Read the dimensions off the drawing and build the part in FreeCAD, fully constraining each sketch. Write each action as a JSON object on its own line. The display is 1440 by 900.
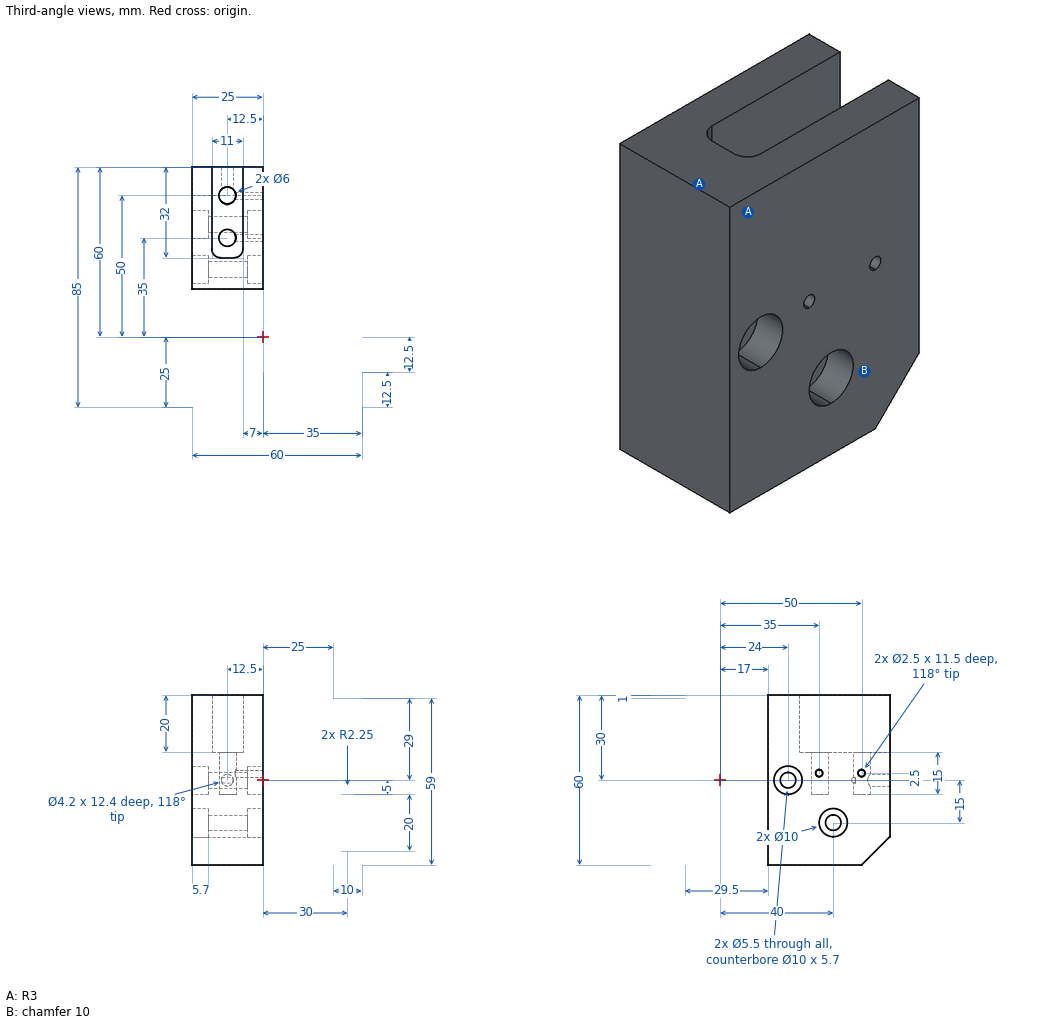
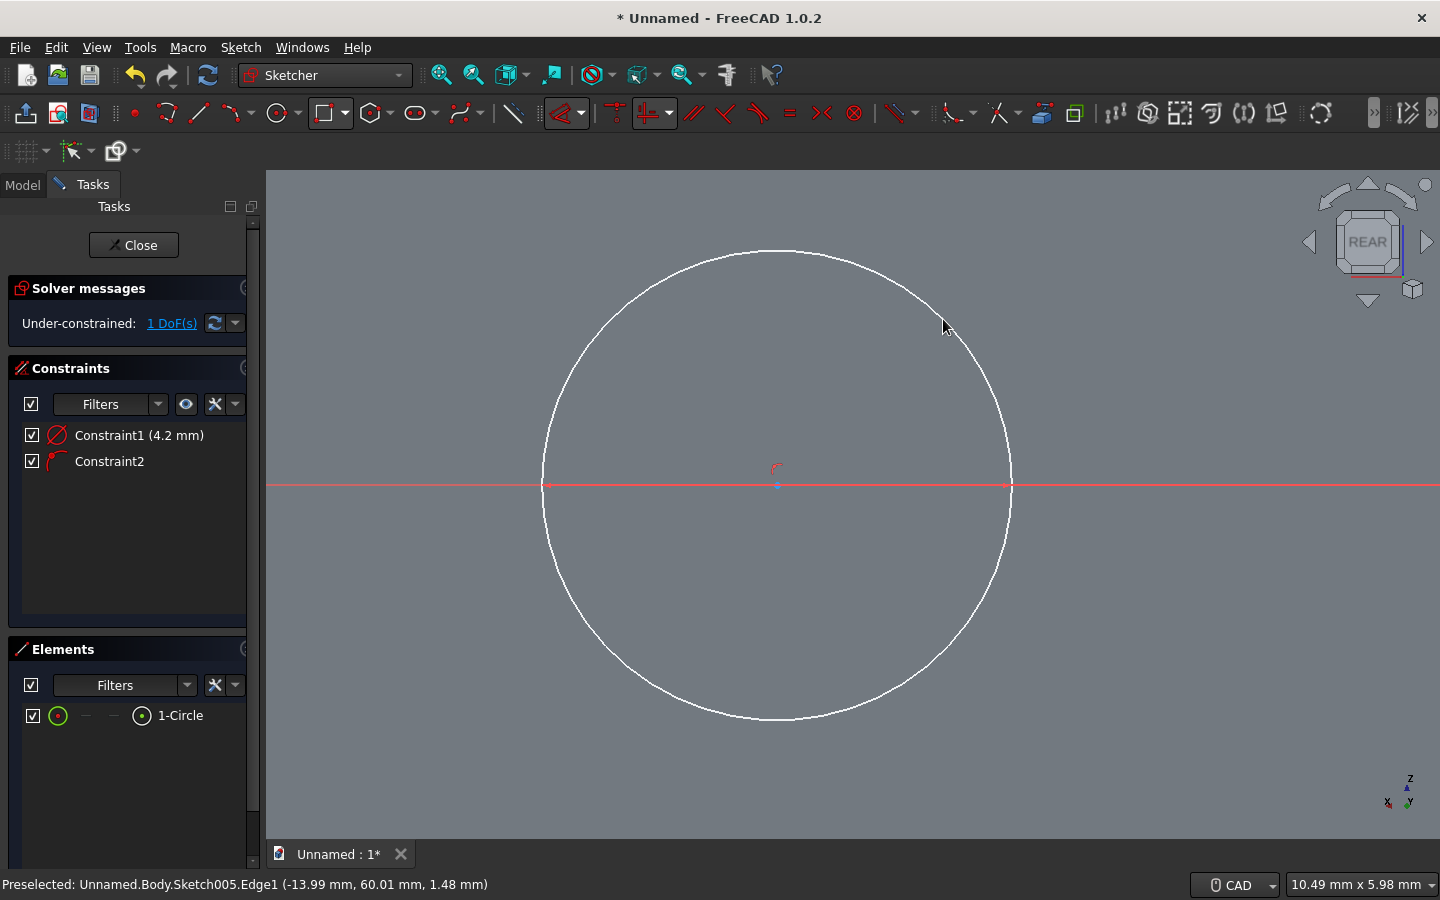
{"action": "left_click", "coordinate": [777, 485]}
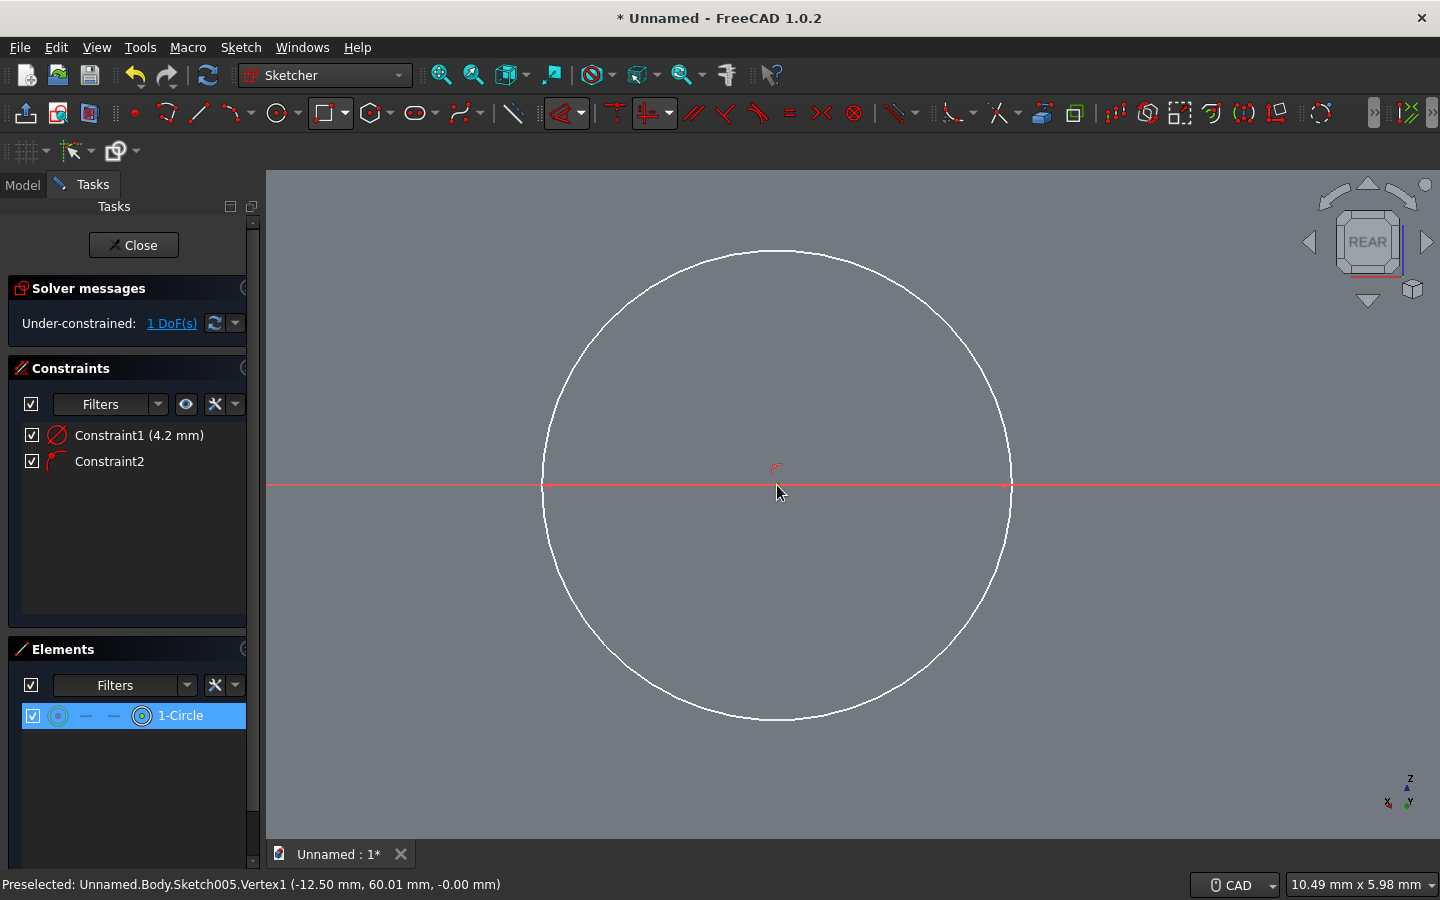
{"action": "left_click", "coordinate": [584, 114]}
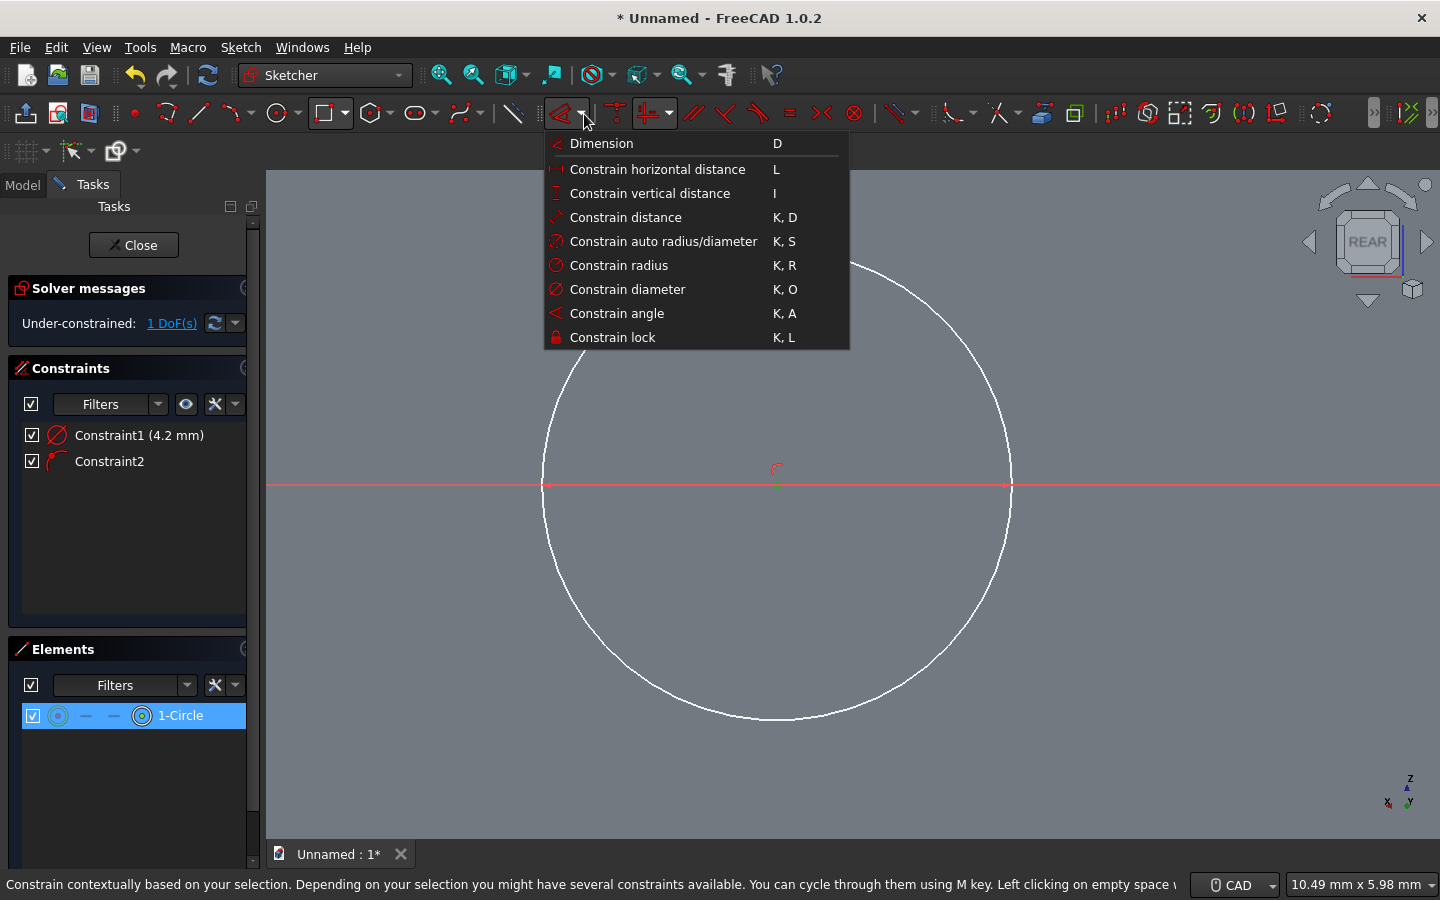
{"action": "left_click", "coordinate": [697, 169]}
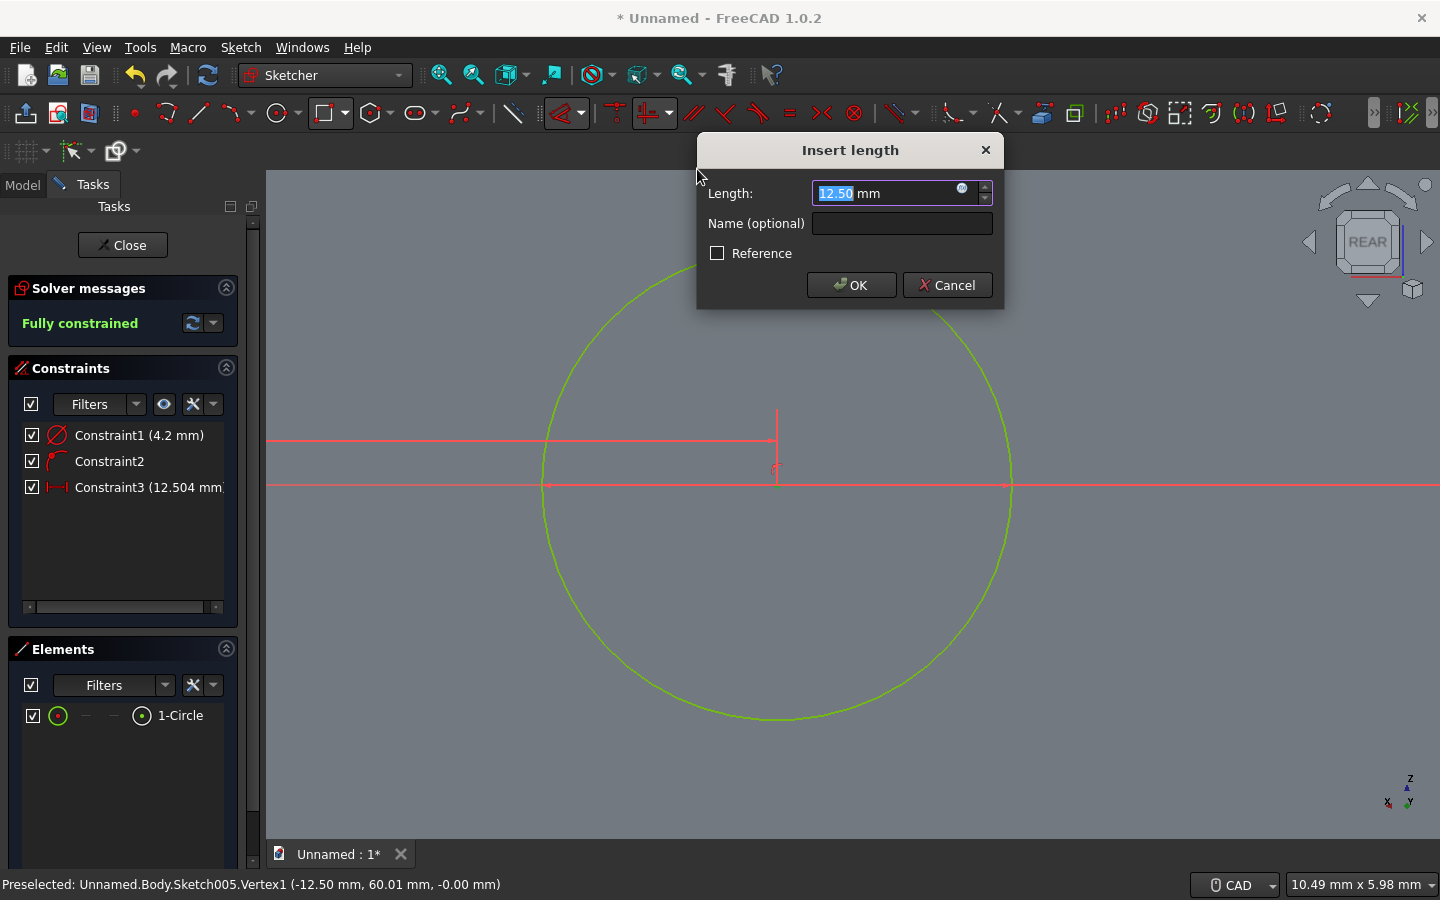
{"action": "type", "text": "12.5"}
{"action": "key", "text": "Return"}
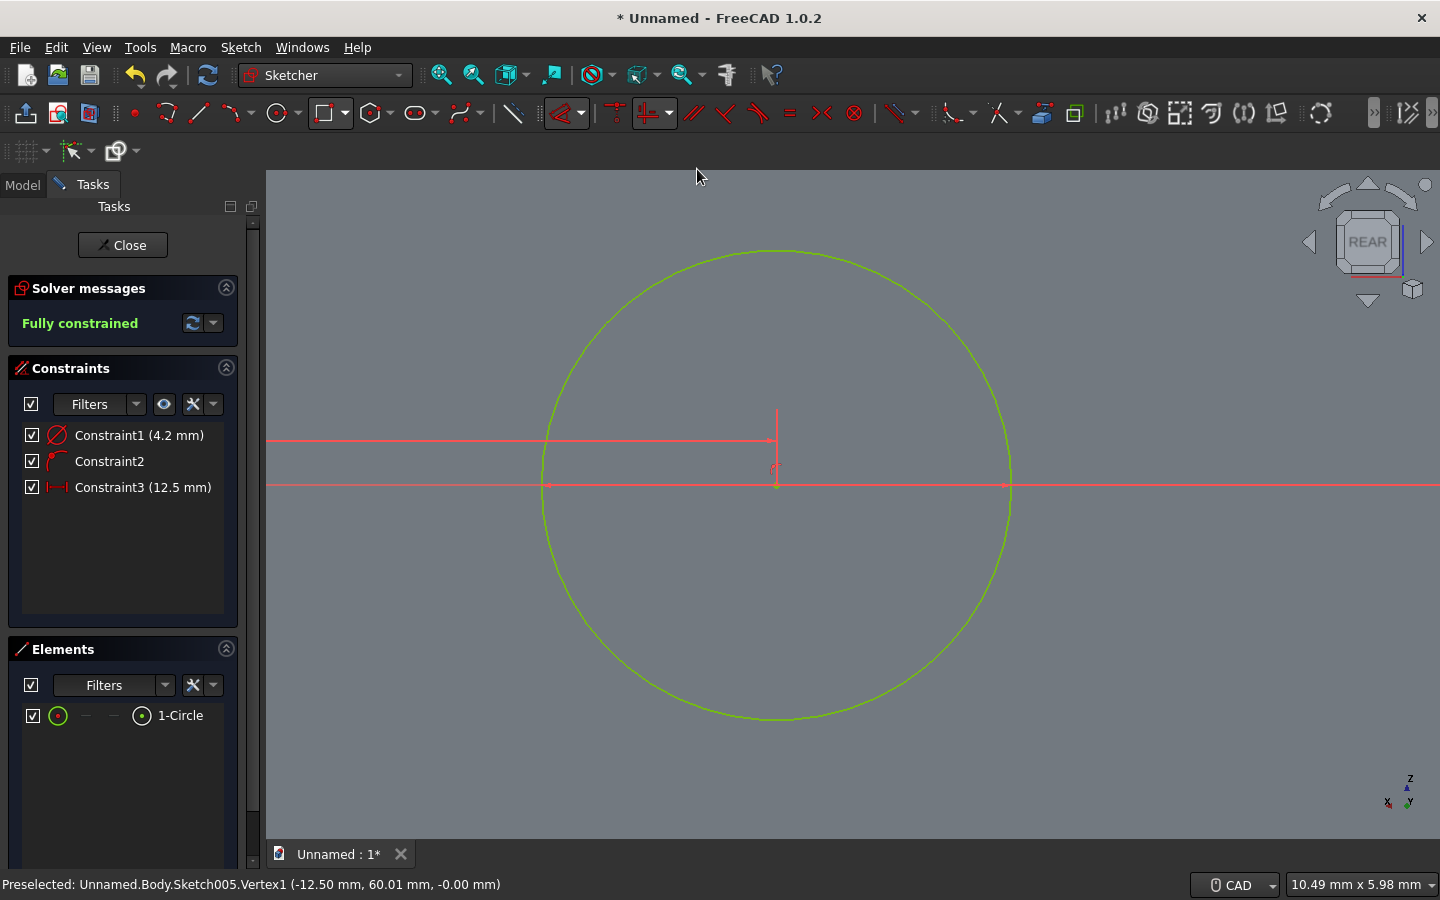
{"action": "left_click", "coordinate": [123, 245]}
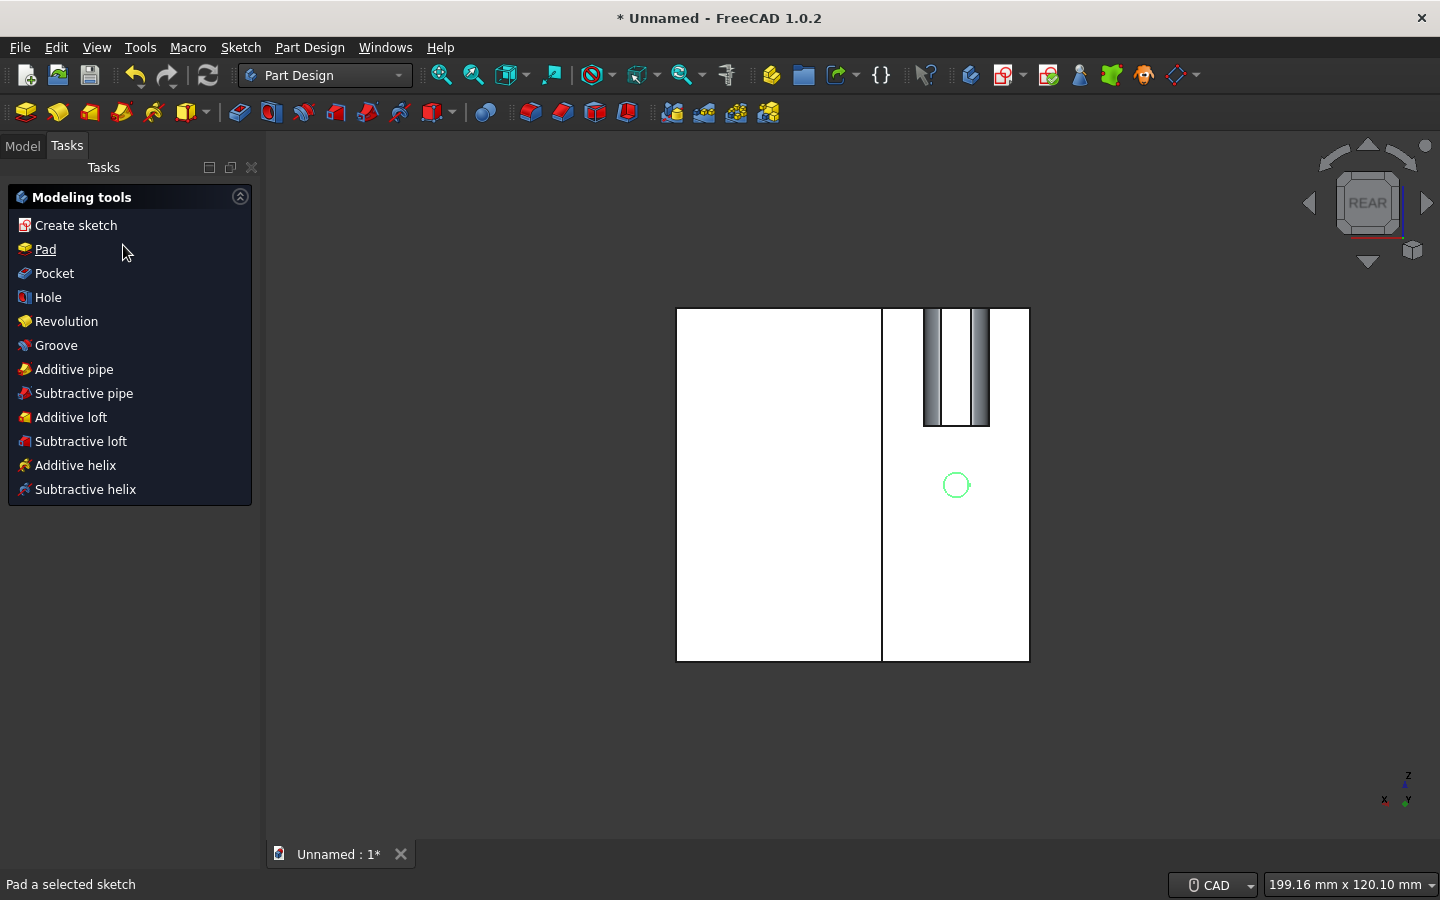
{"action": "left_click", "coordinate": [272, 112]}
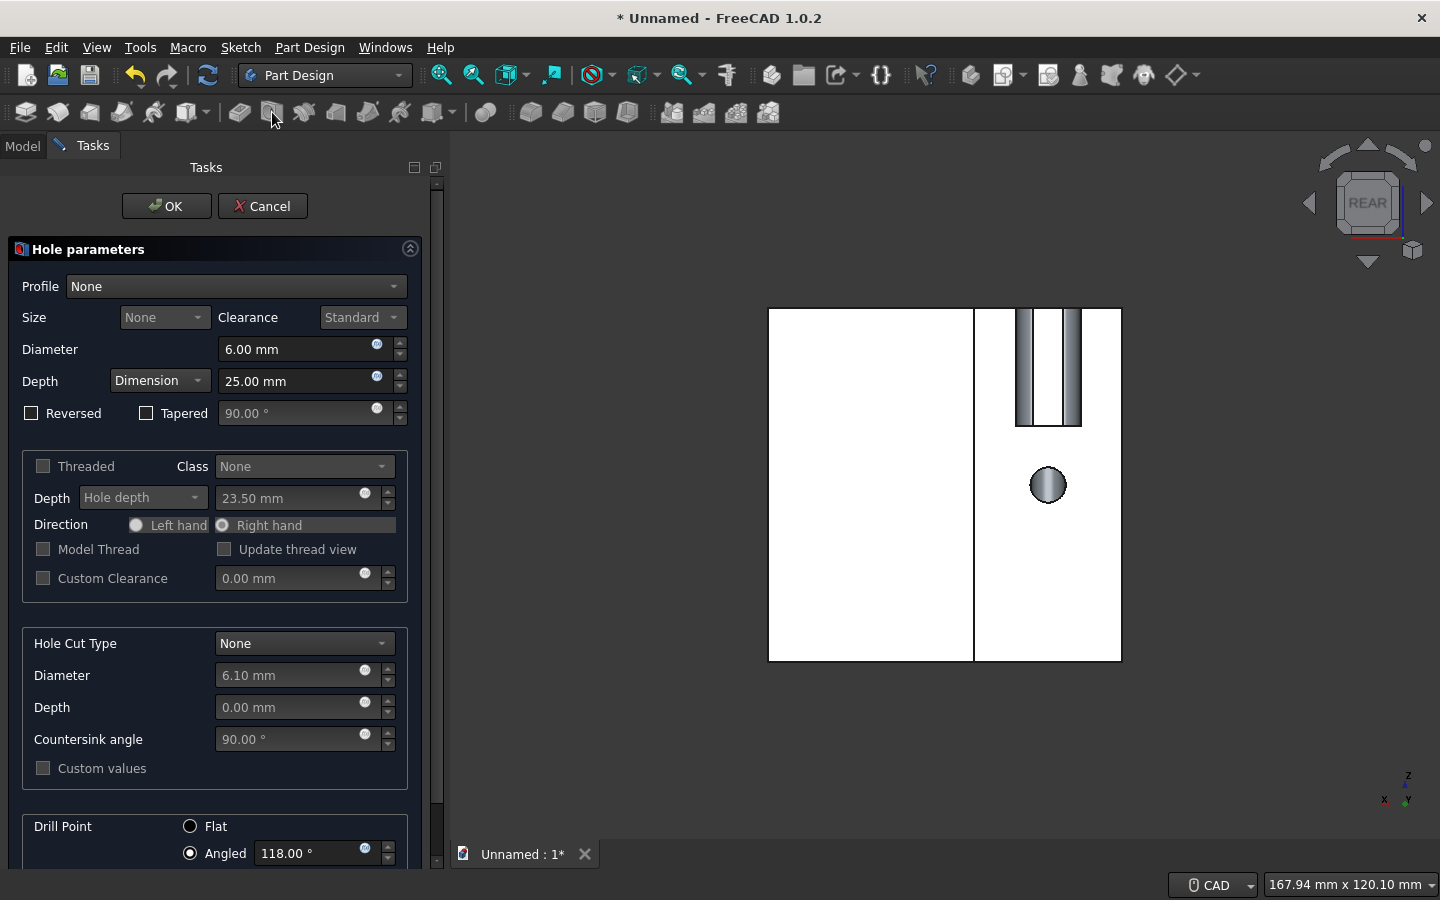
{"action": "triple_click", "coordinate": [305, 349]}